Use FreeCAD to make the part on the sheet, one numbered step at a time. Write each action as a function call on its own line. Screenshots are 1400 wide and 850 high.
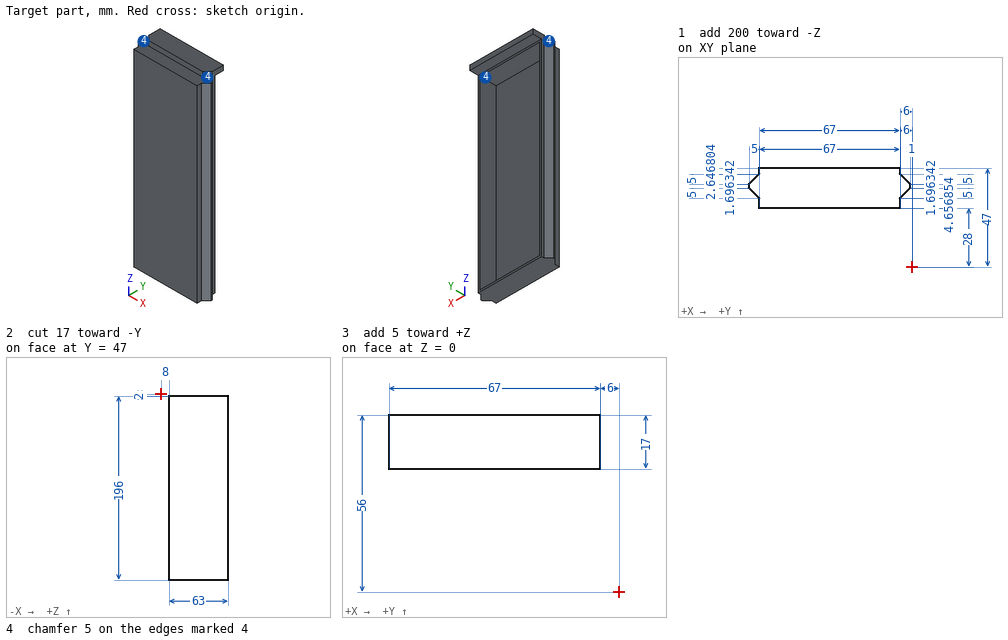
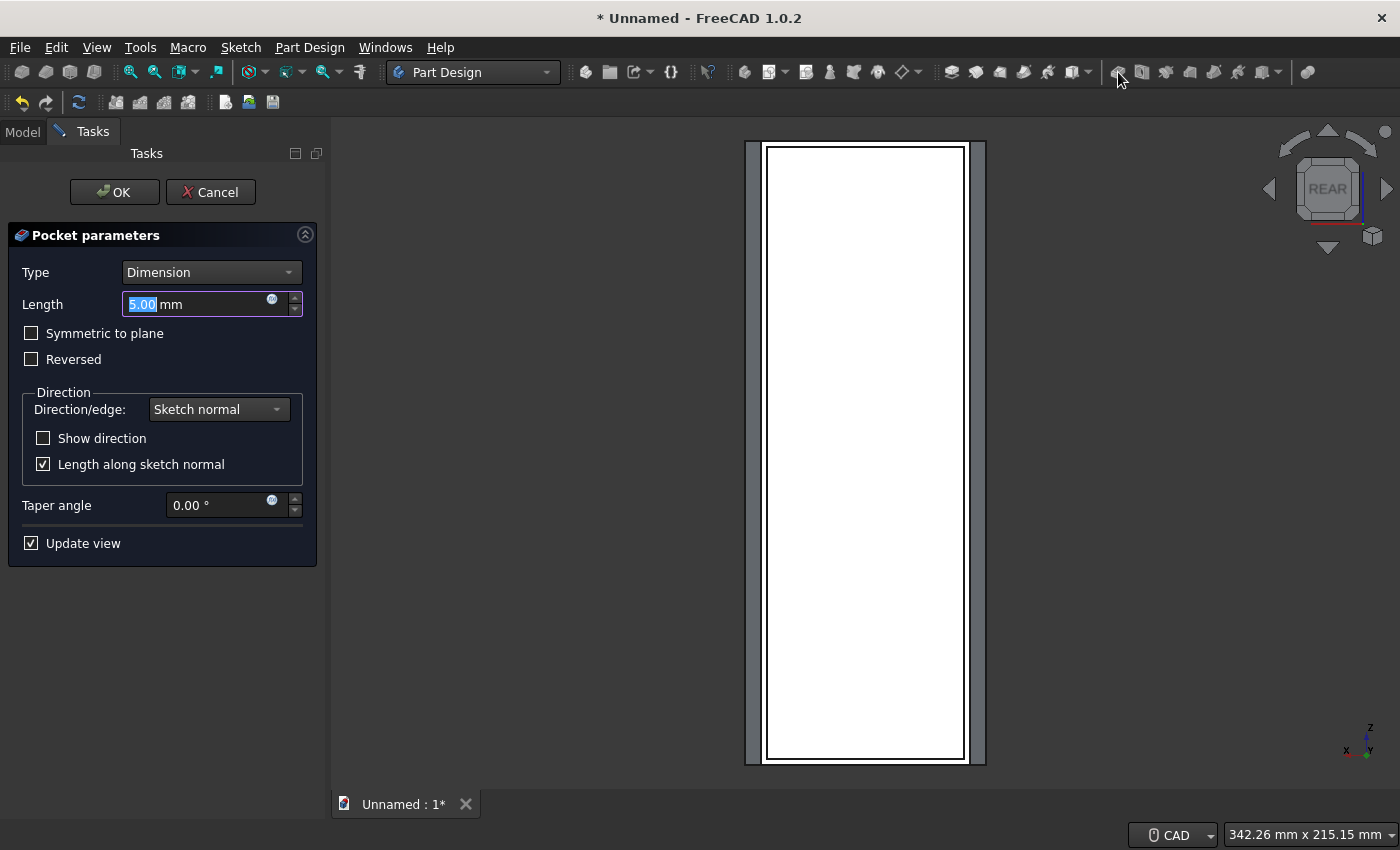
text(17)
key(Tab)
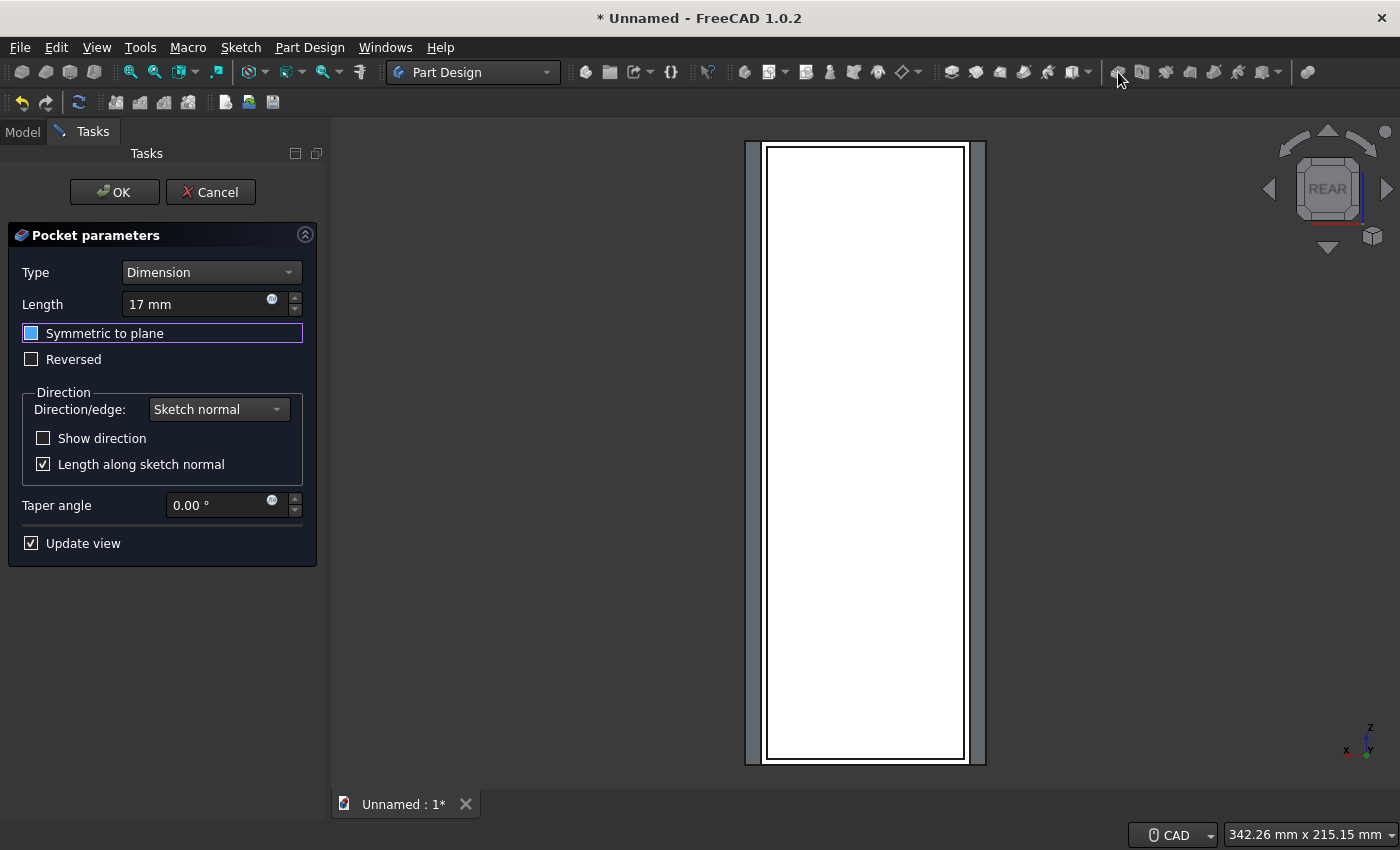
click(115, 192)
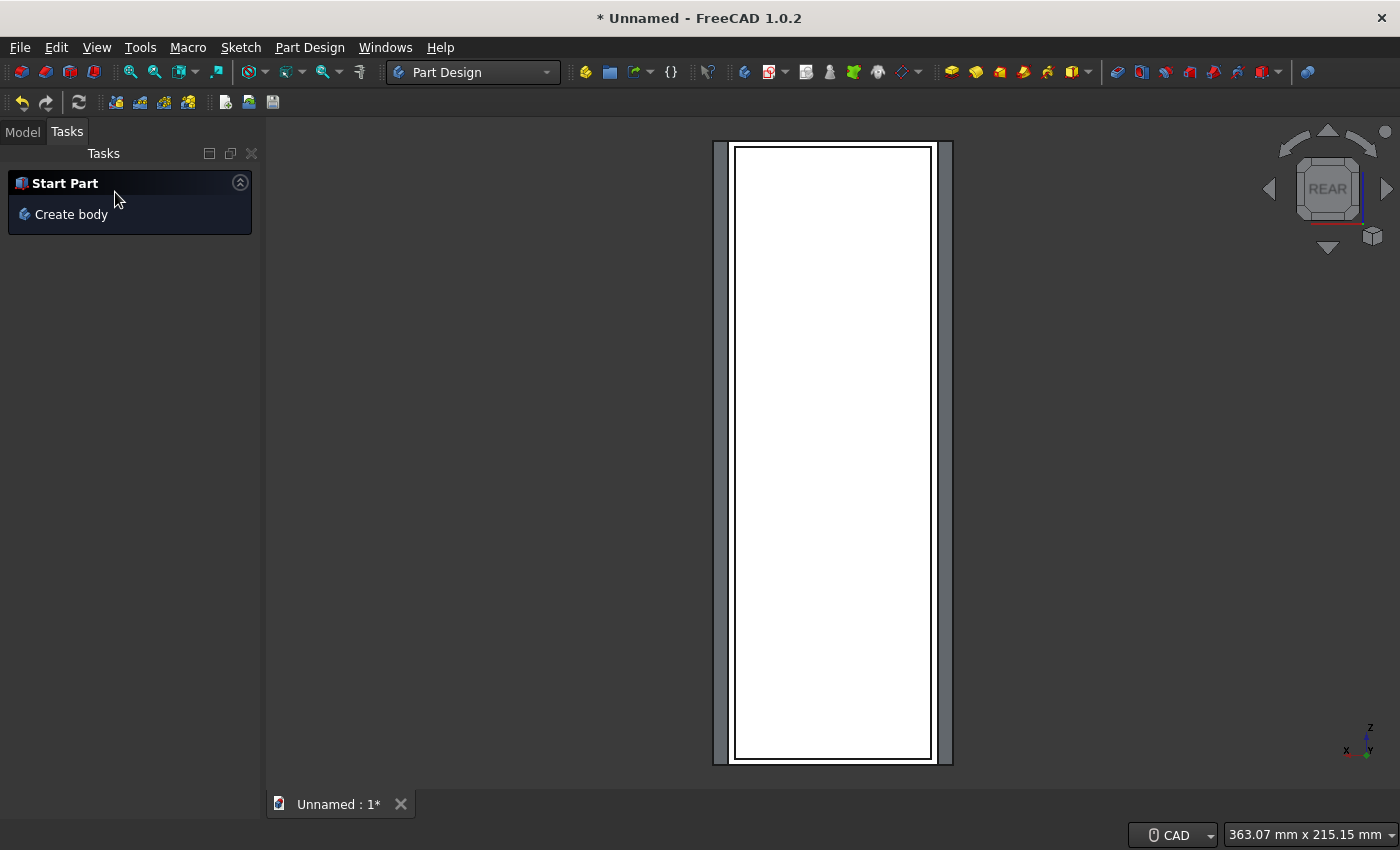
key(0)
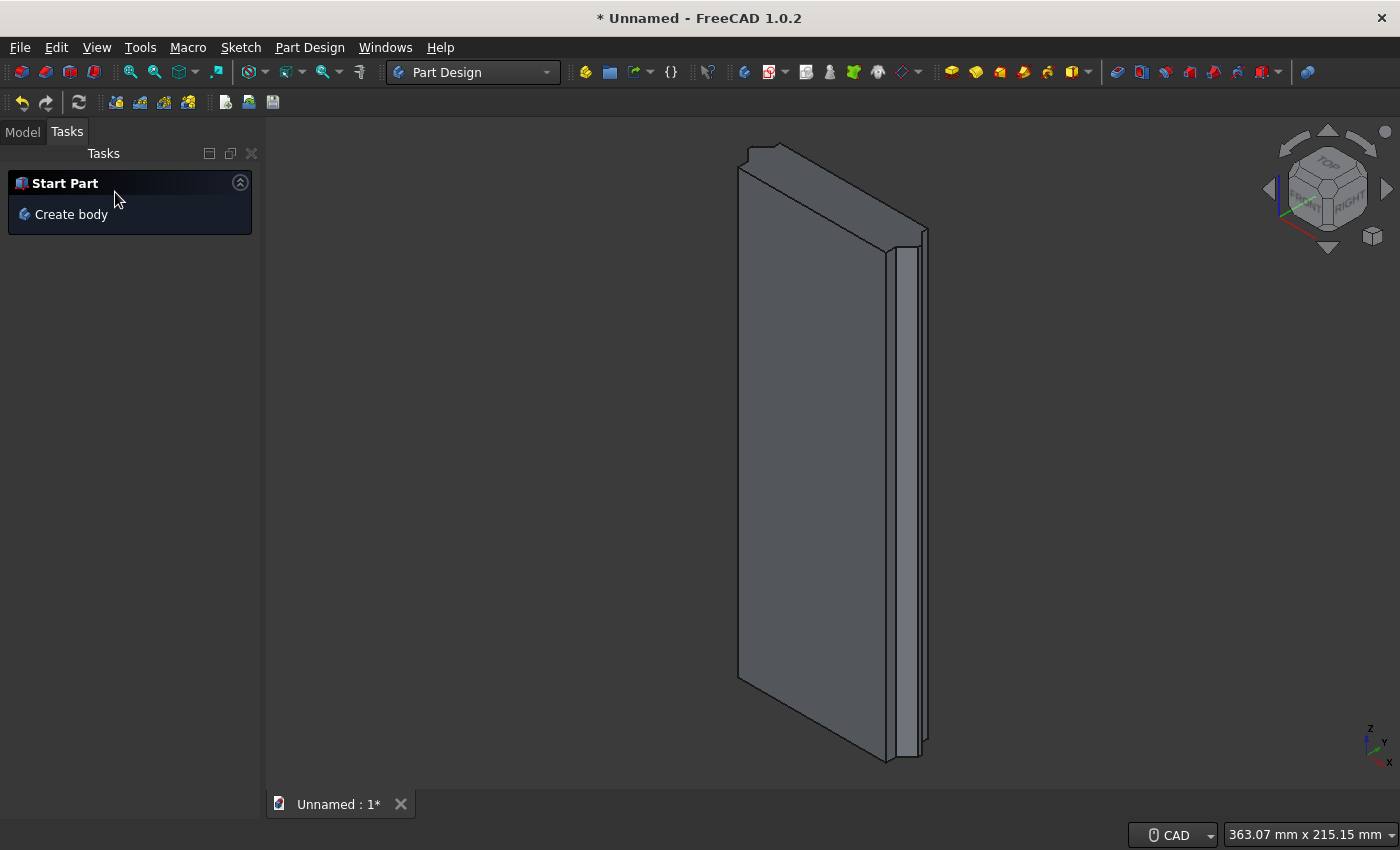
click(882, 225)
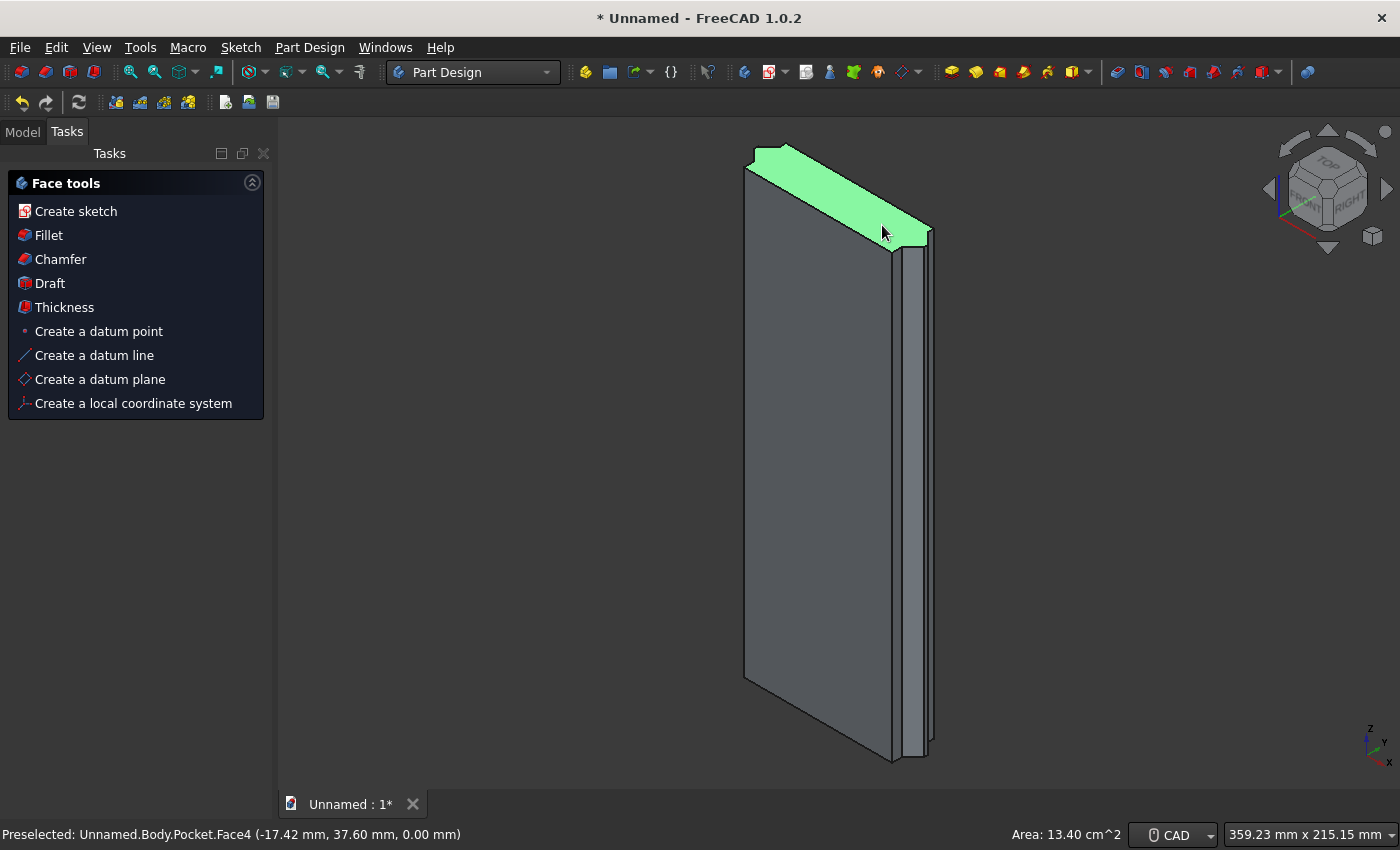
click(770, 72)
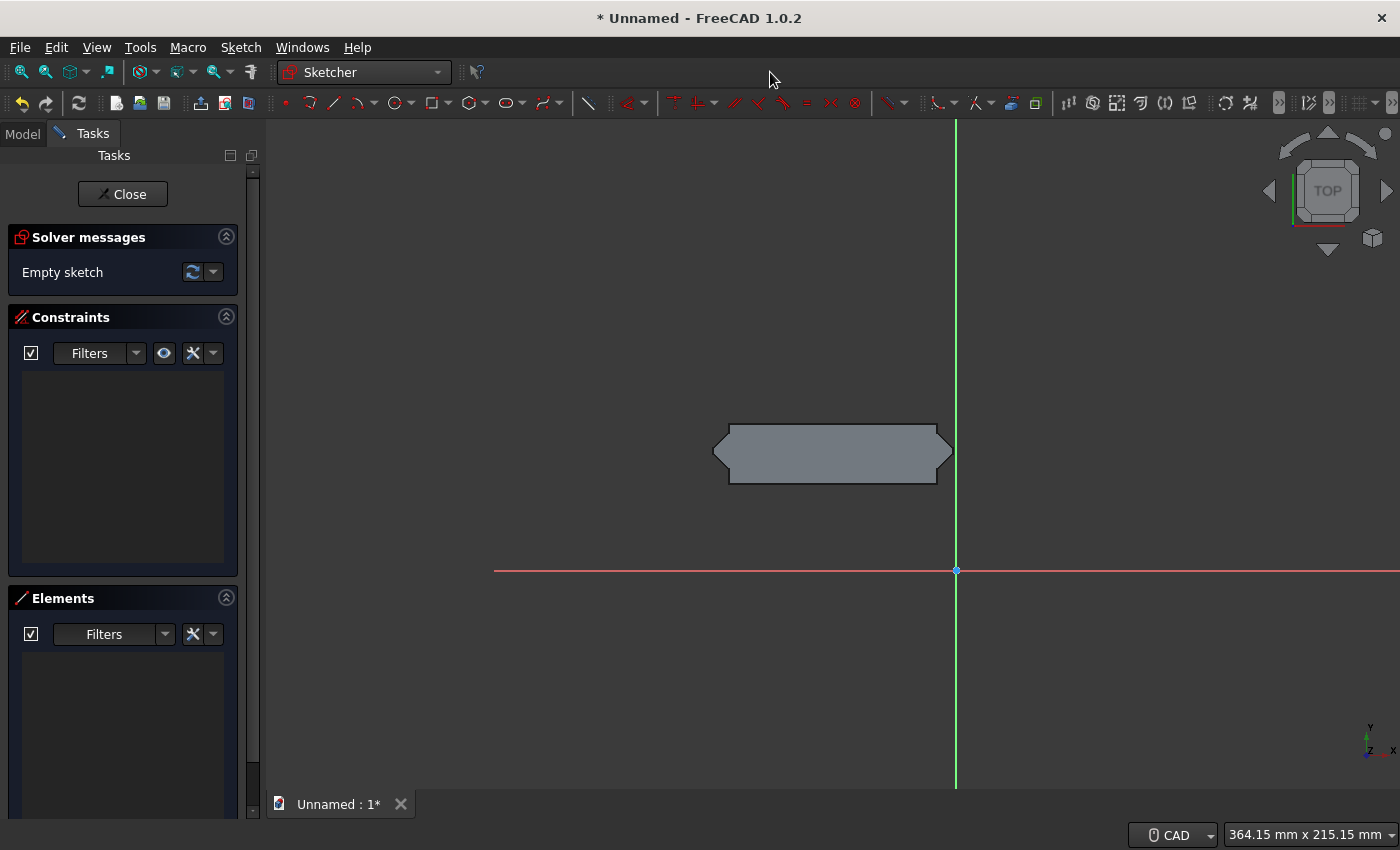
scroll(888, 501, up, 5)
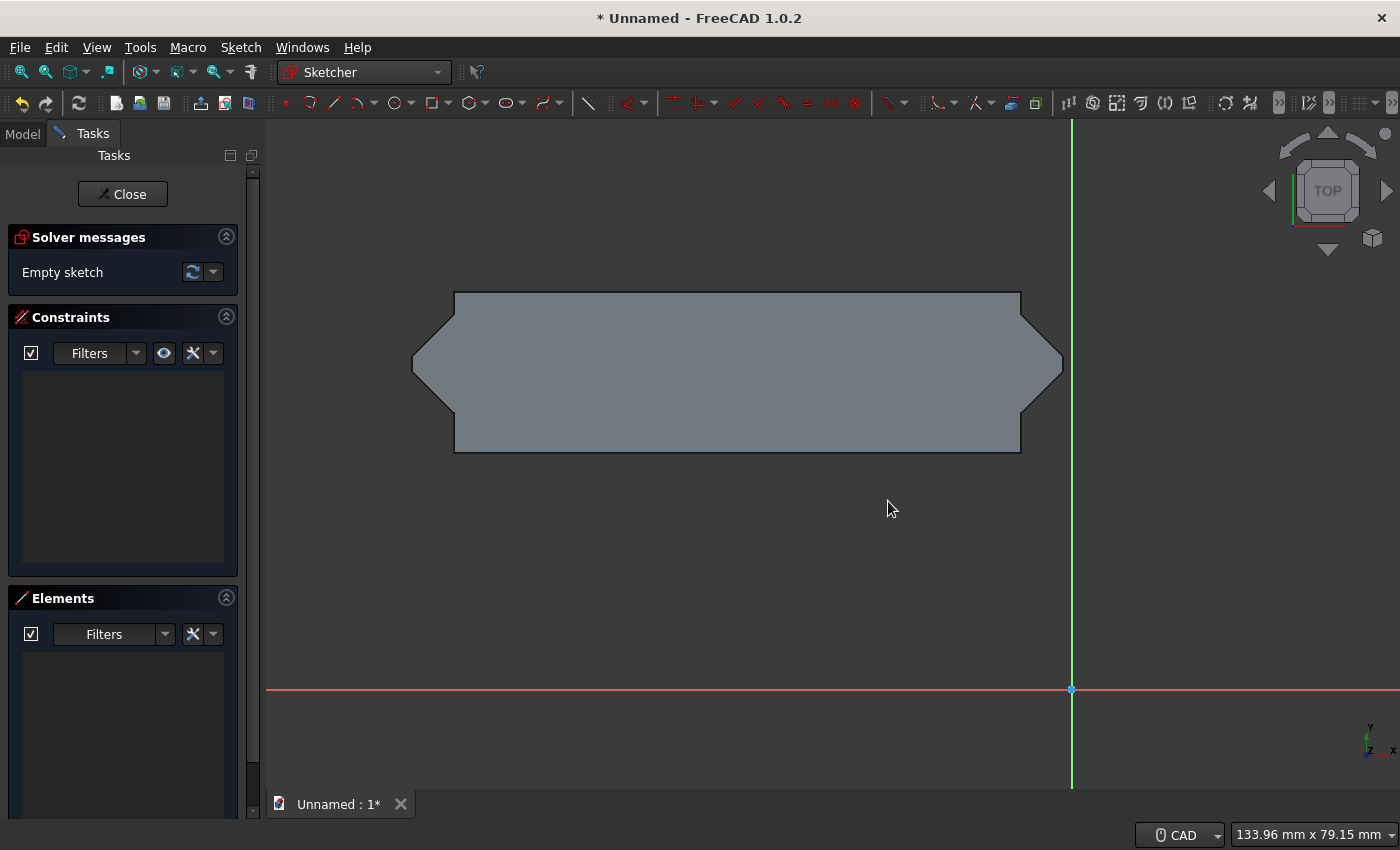
key(g)
key(r)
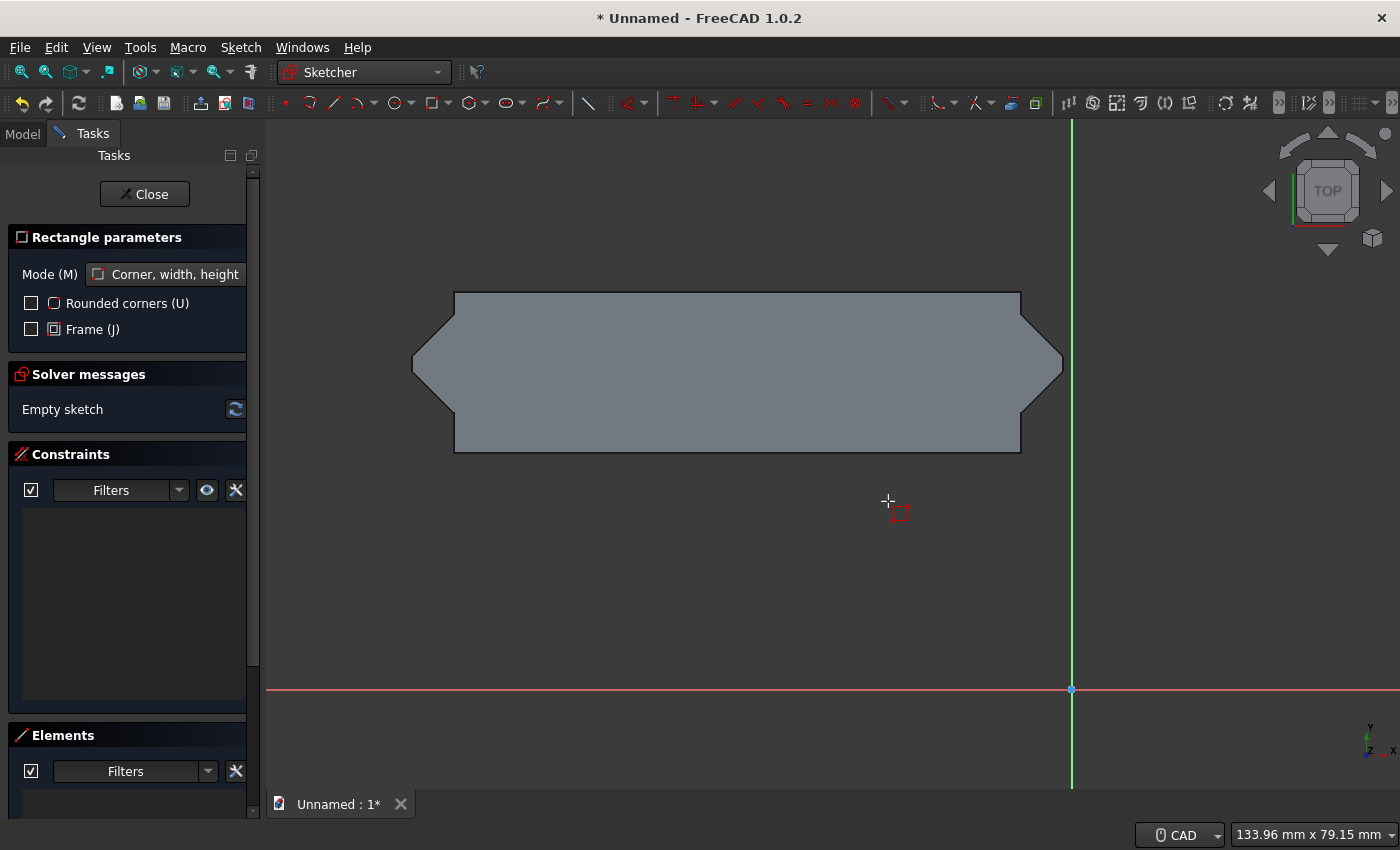
click(454, 216)
move(1021, 360)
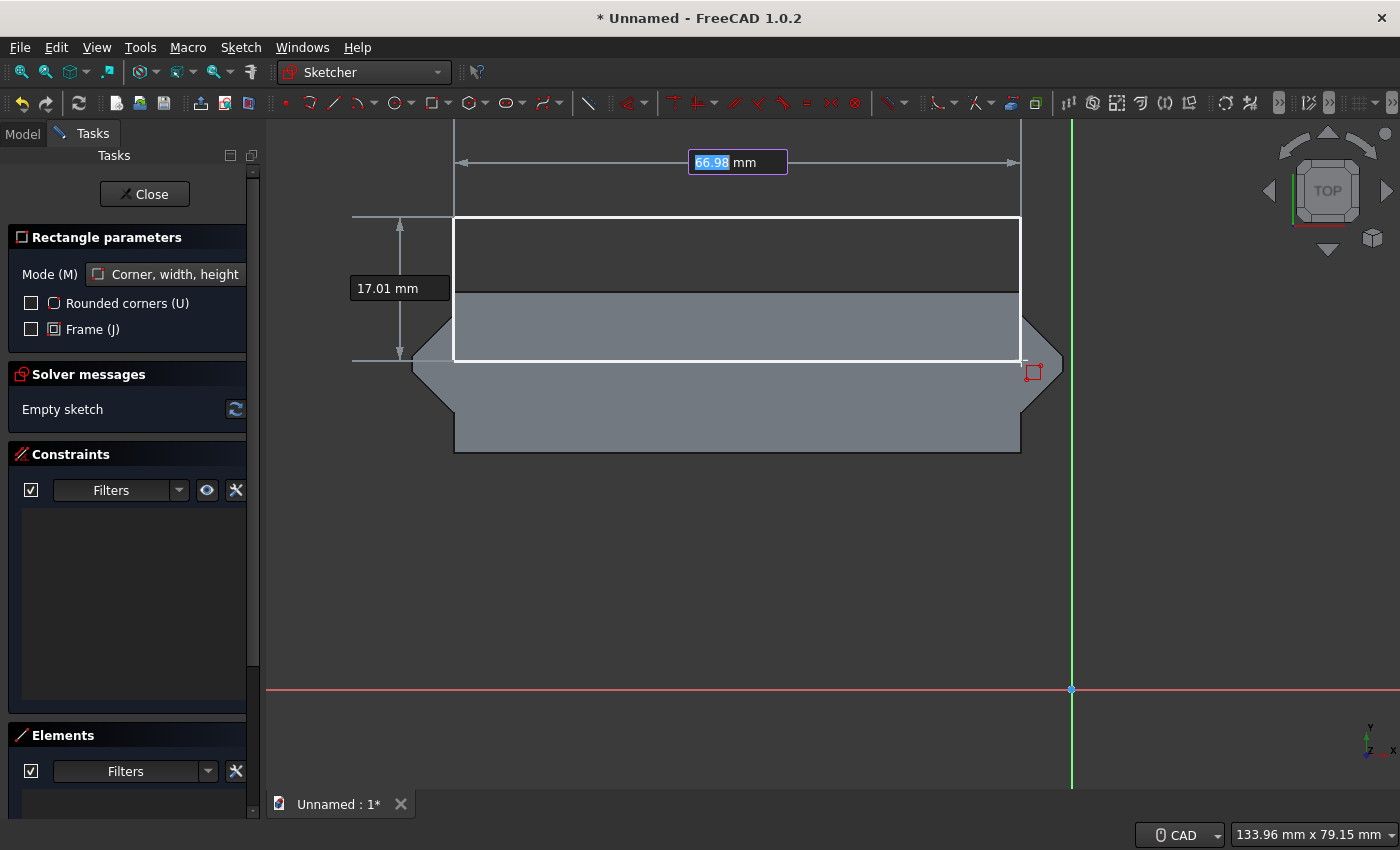
text(67)
key(Tab)
text(17)
key(Return)
key(Escape)